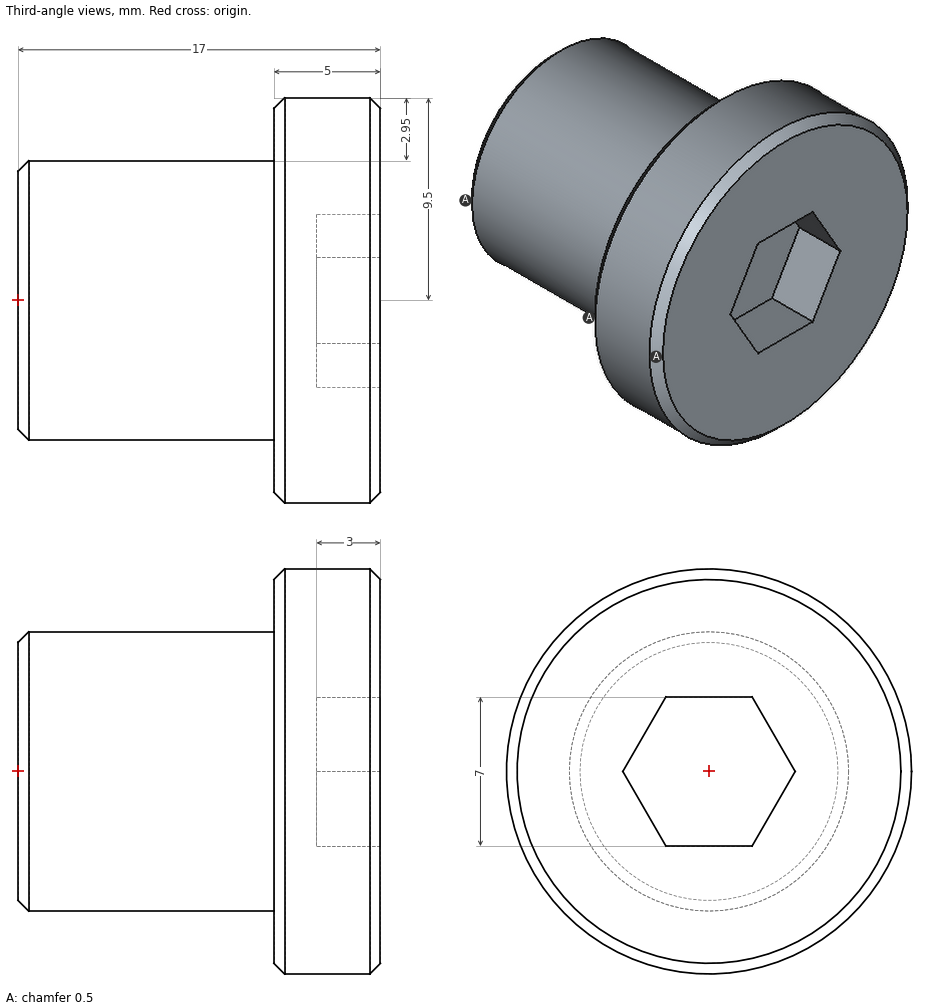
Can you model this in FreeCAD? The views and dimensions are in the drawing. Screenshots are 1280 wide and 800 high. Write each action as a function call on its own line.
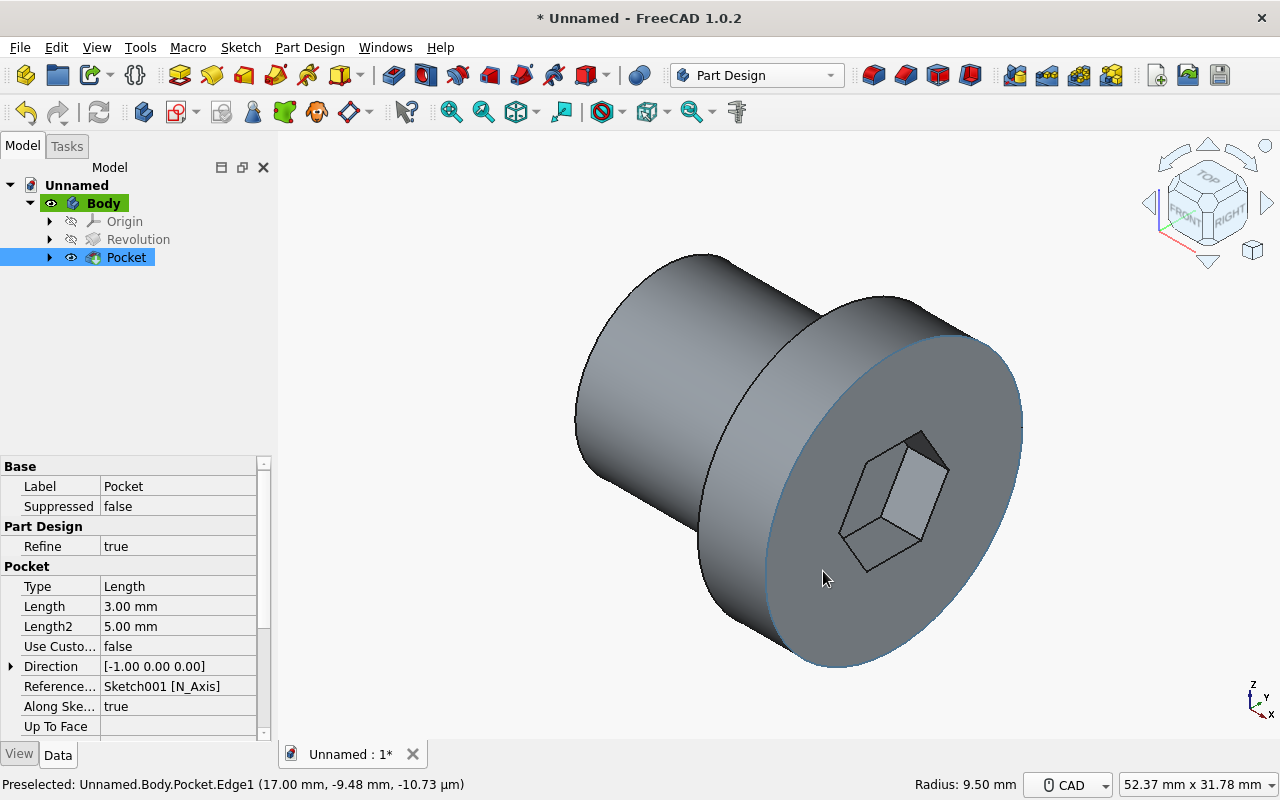
key(2)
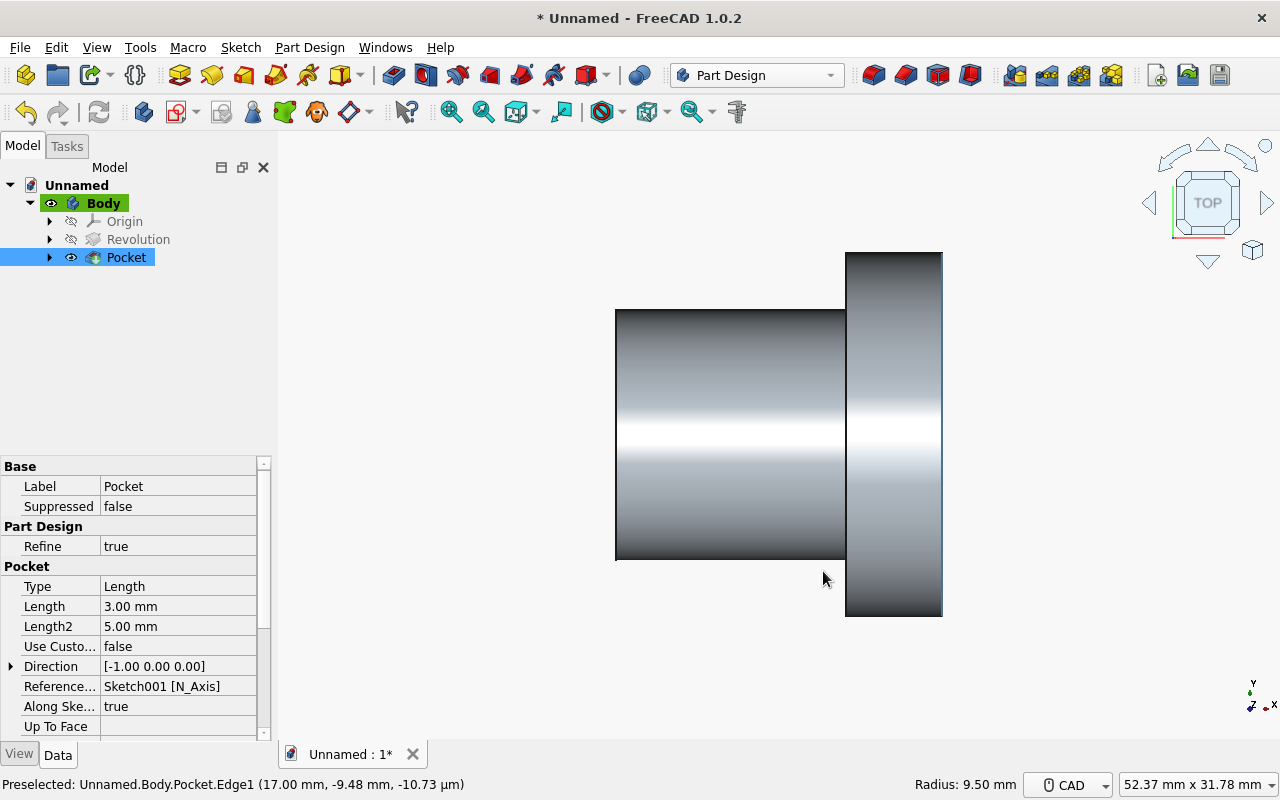
click(846, 581, ctrl)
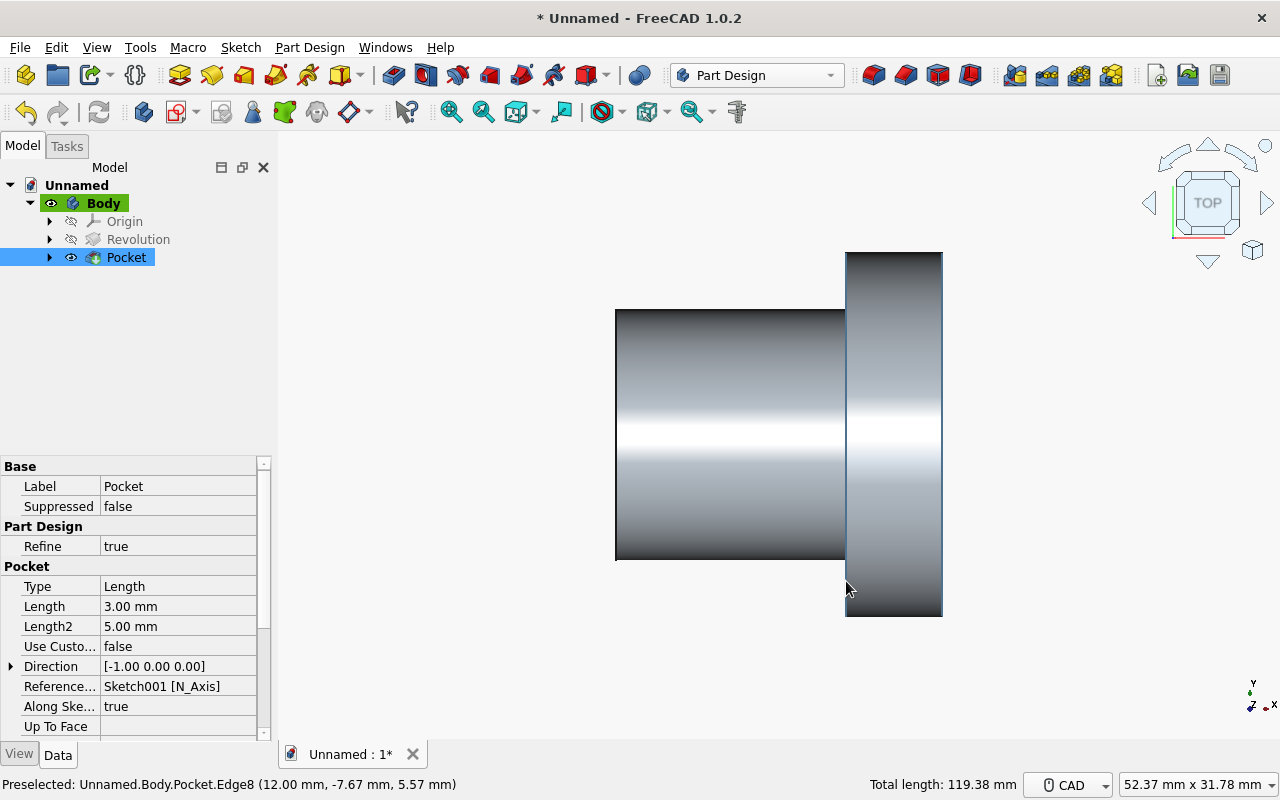
click(616, 536, ctrl)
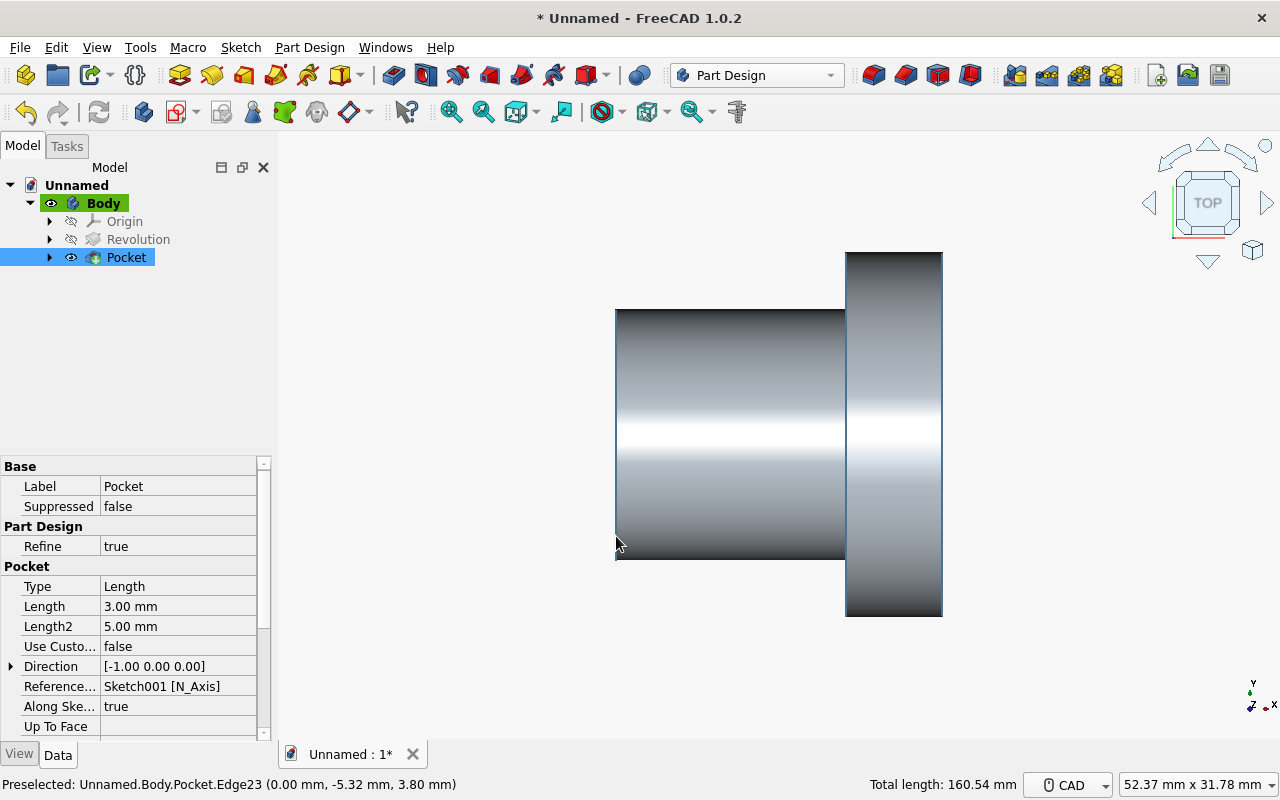
click(906, 76)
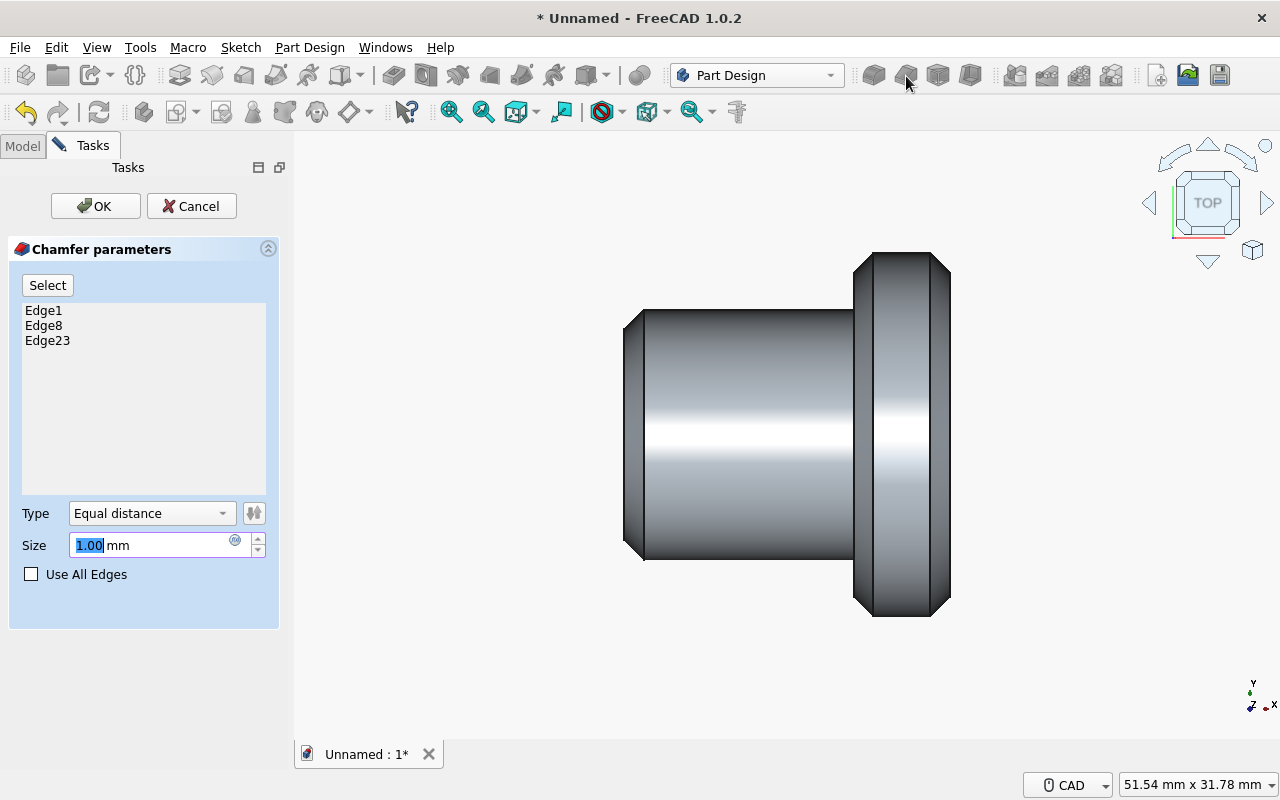
text(0.5)
key(Tab)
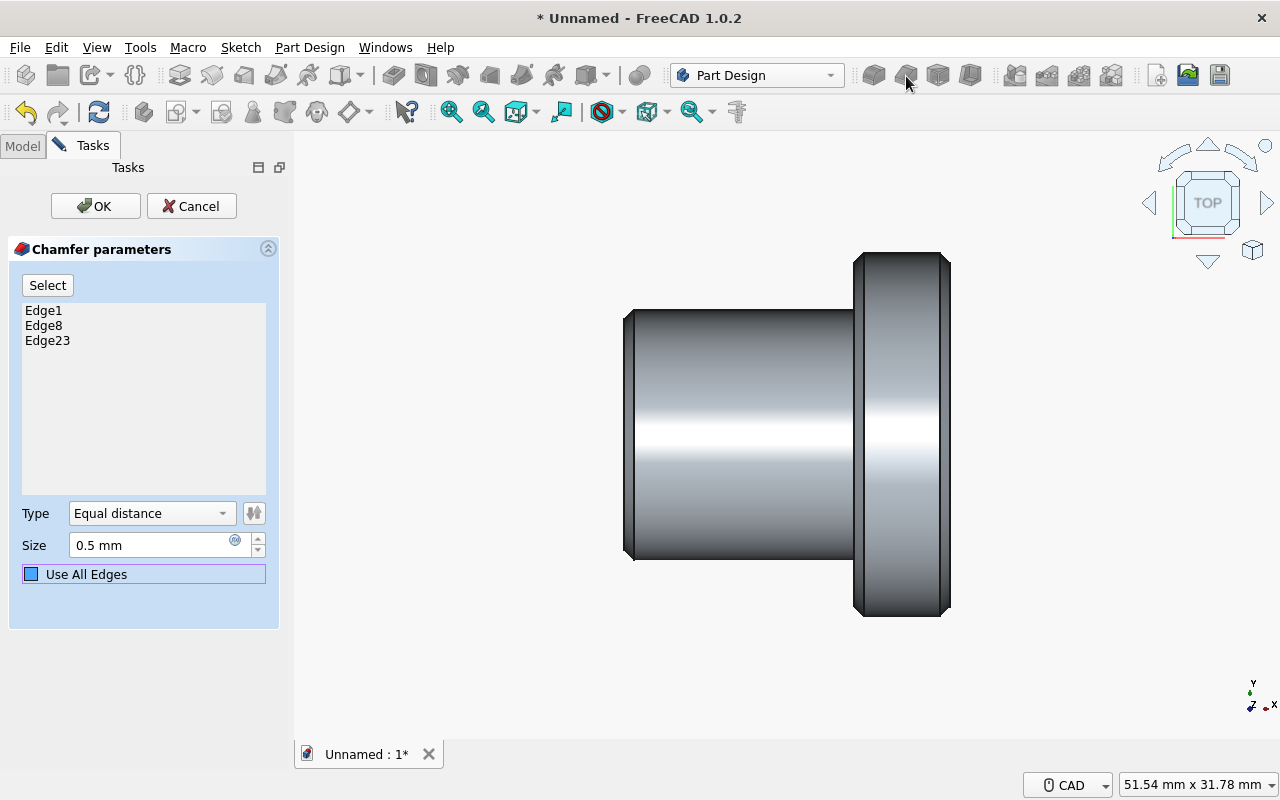
click(96, 206)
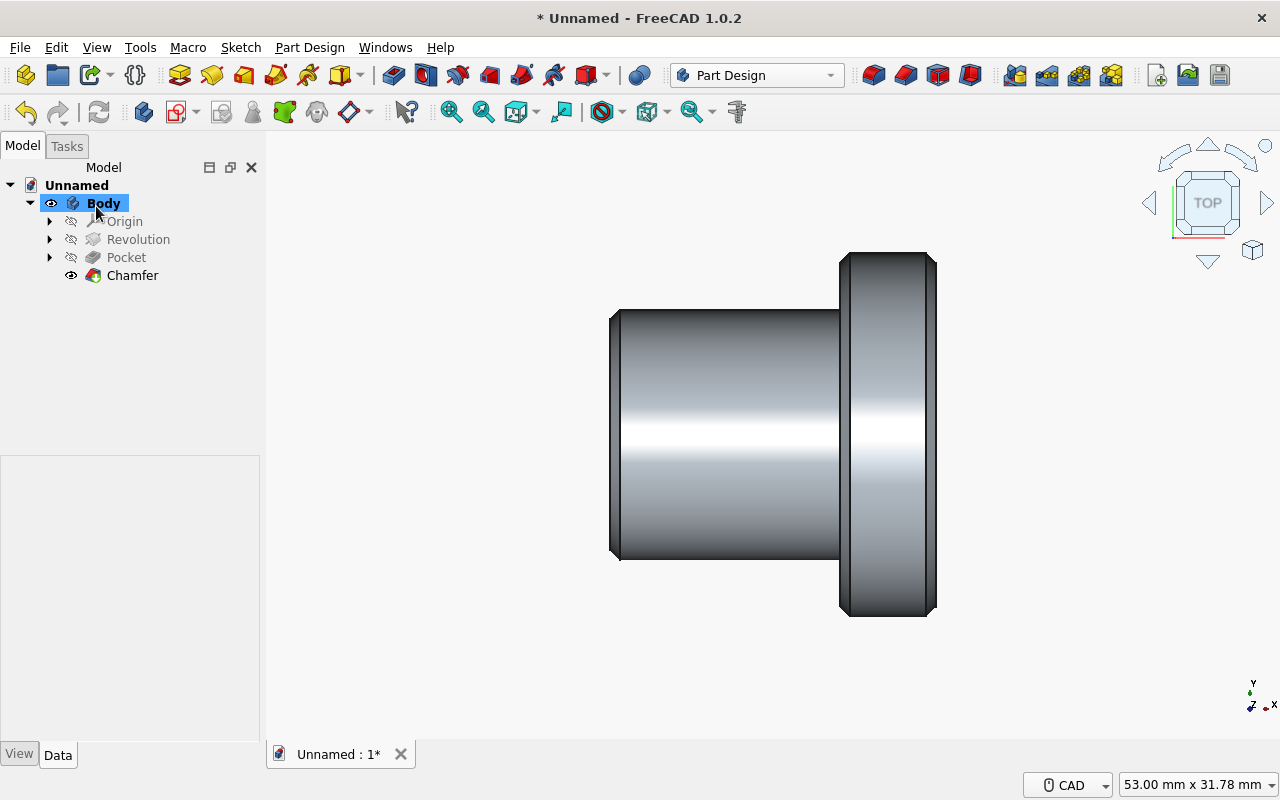
key(0)